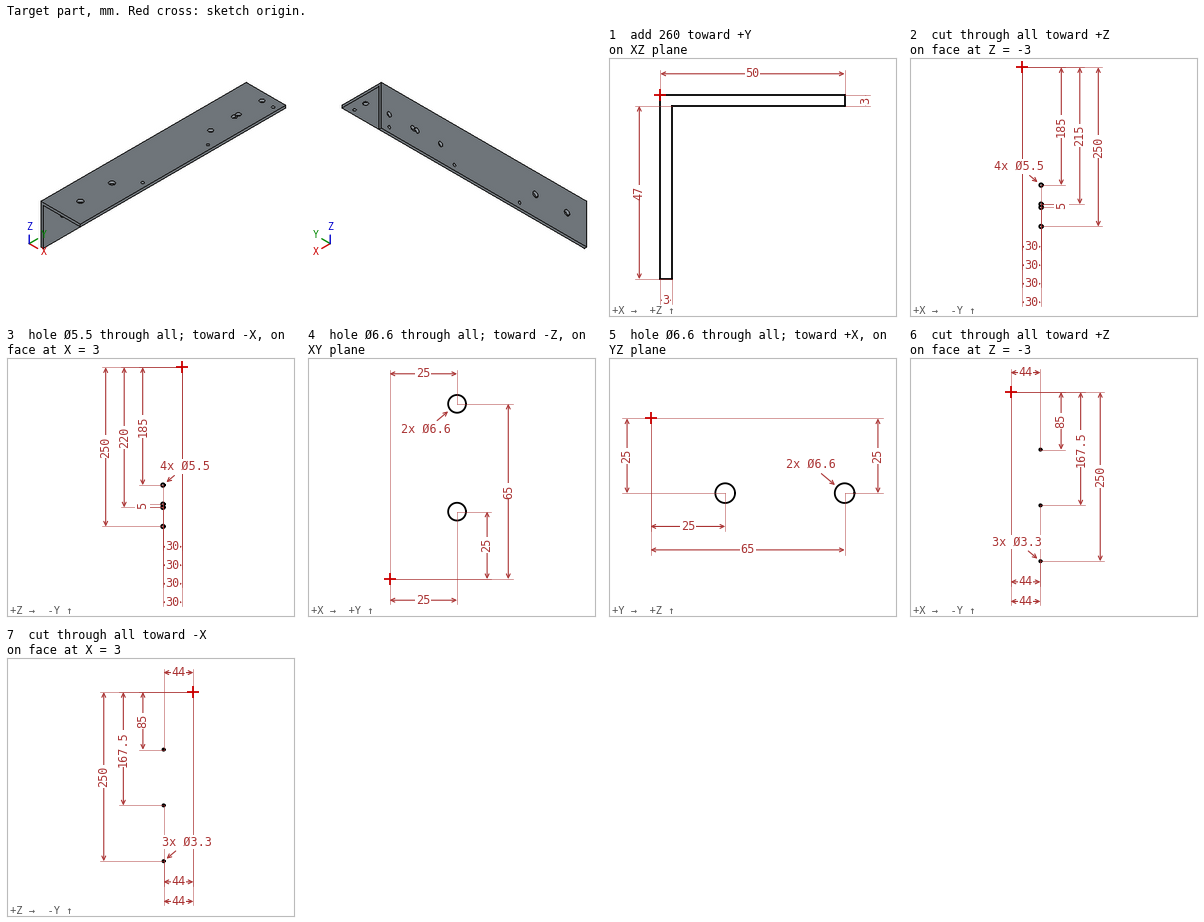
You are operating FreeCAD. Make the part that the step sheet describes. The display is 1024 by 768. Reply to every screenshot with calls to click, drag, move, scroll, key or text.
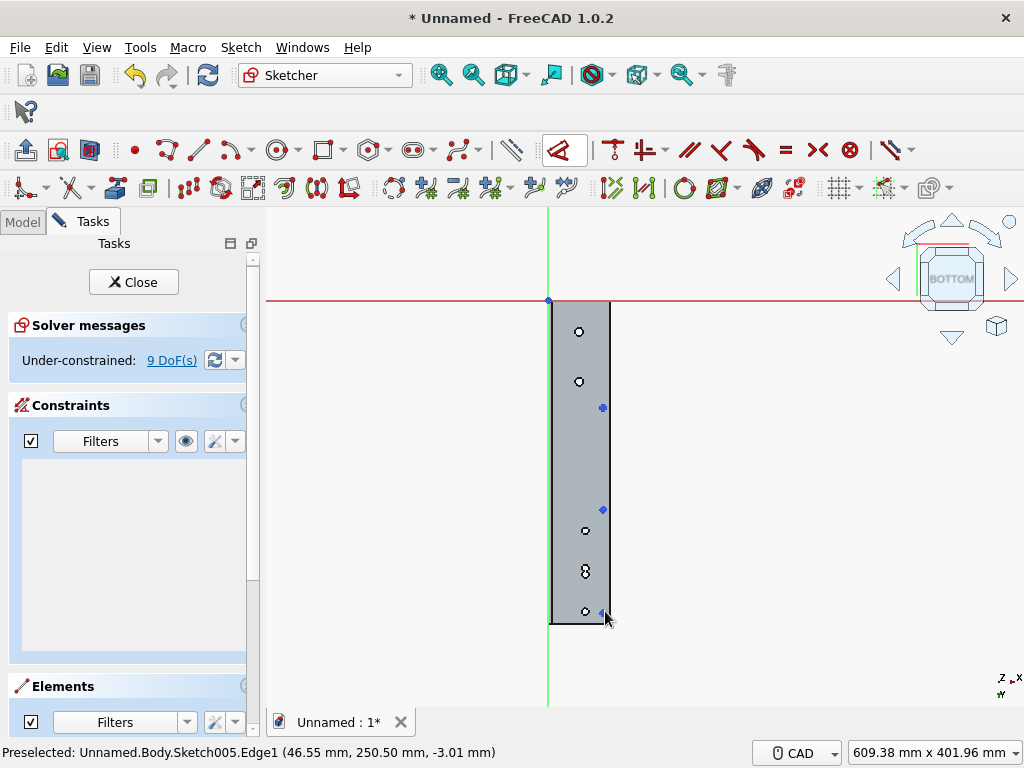
scroll(605, 508, up, 9)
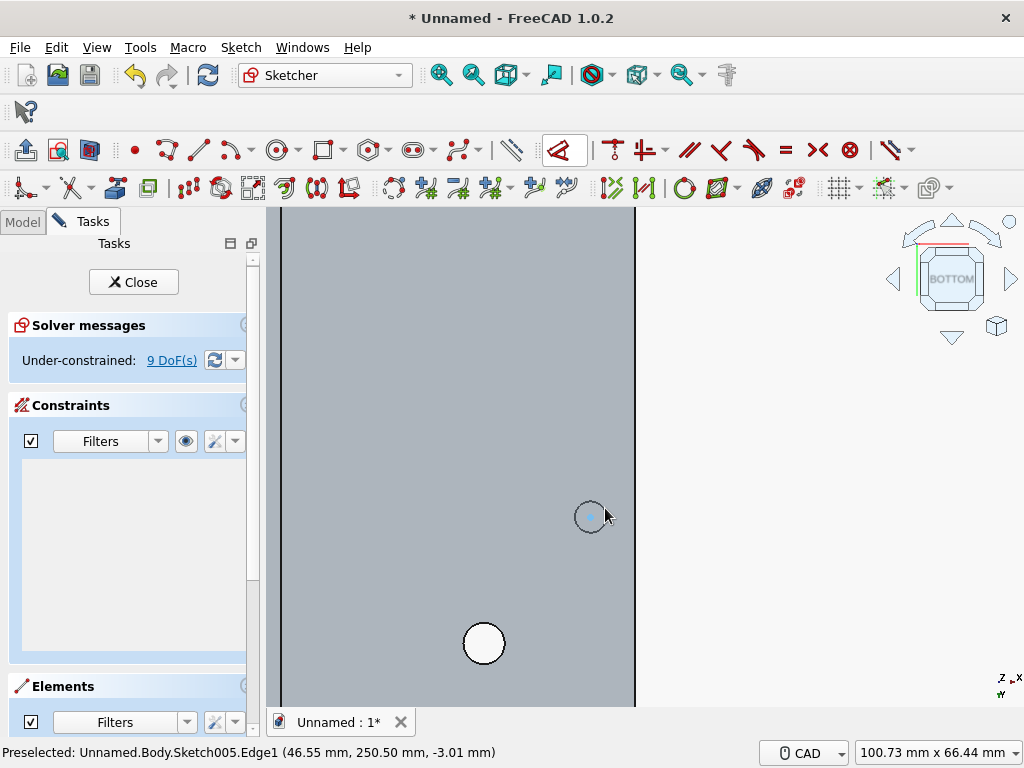
click(602, 506)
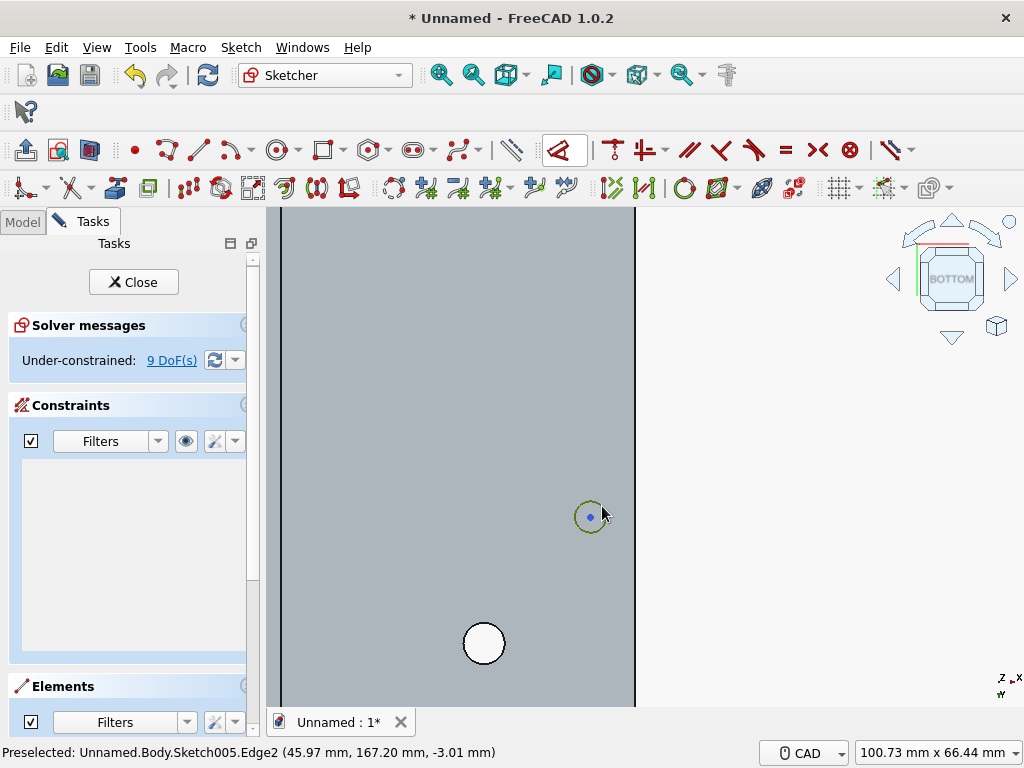
scroll(605, 508, down, 9)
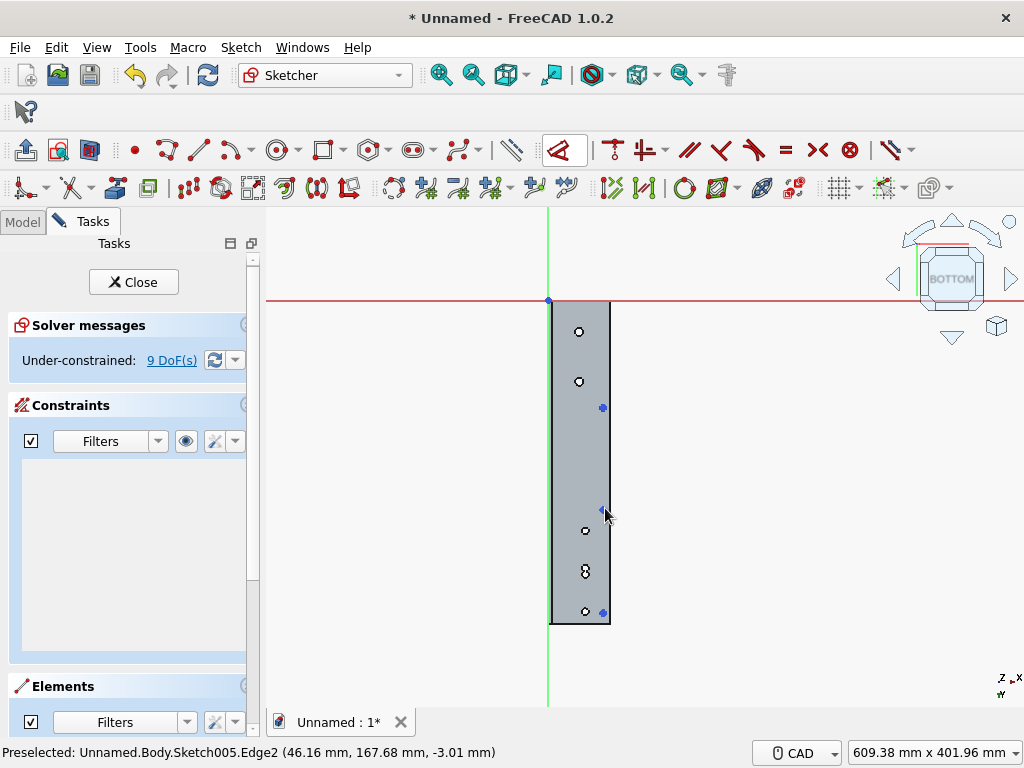
scroll(605, 406, up, 8)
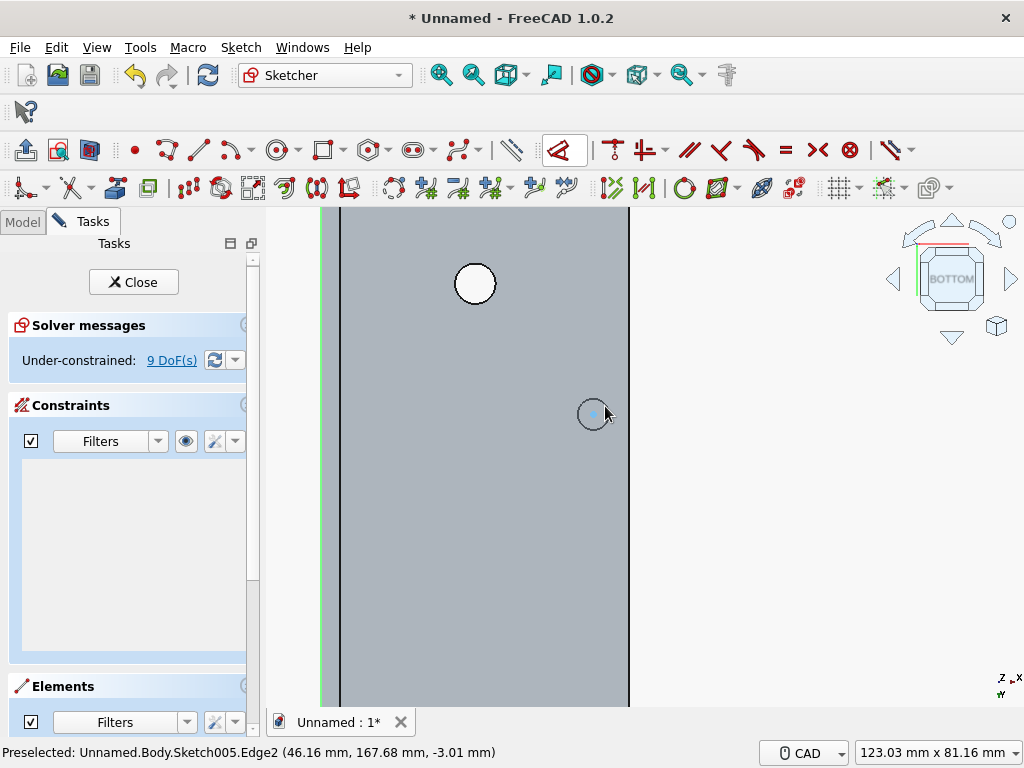
click(604, 403)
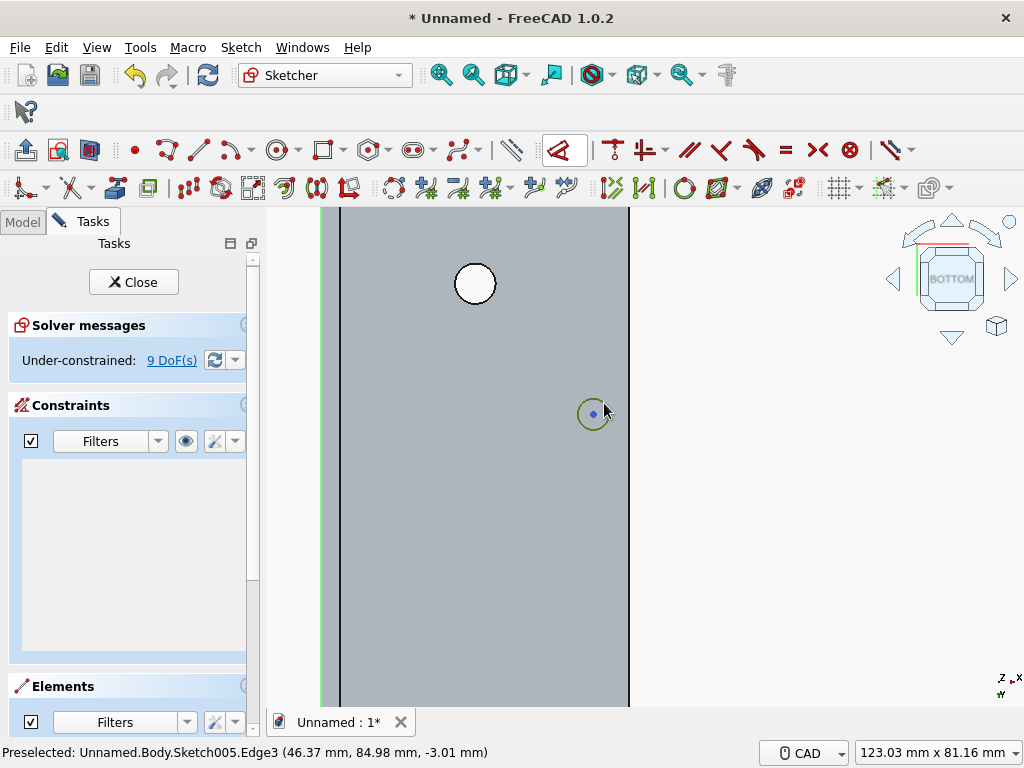
click(786, 150)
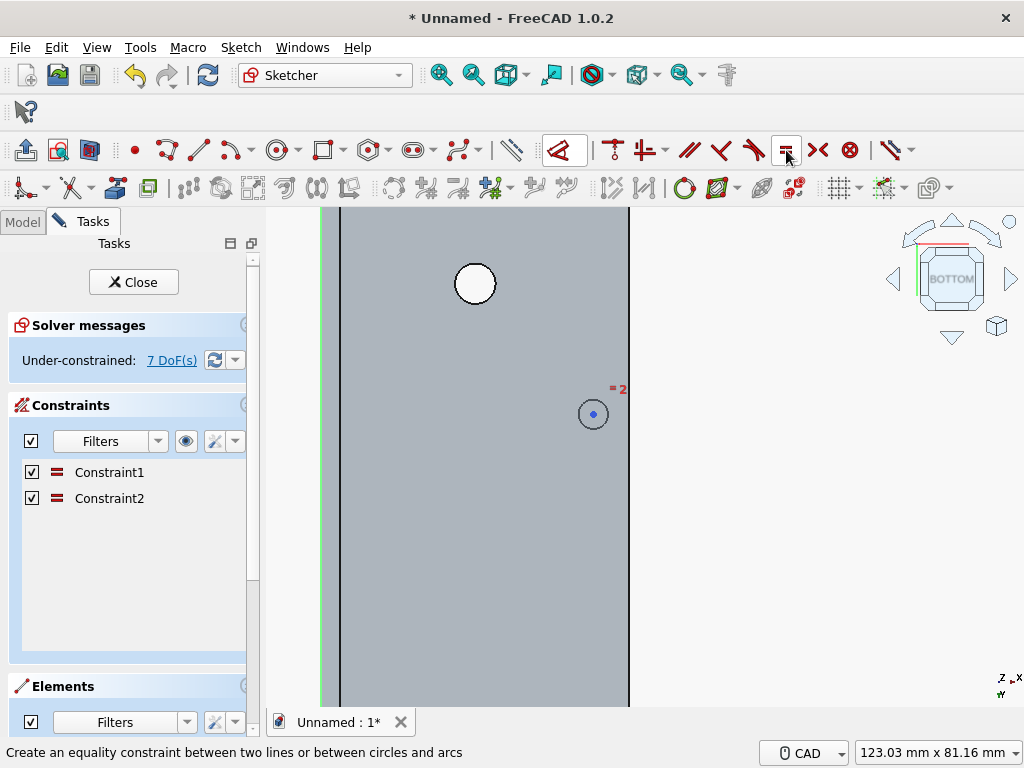
scroll(605, 406, down, 8)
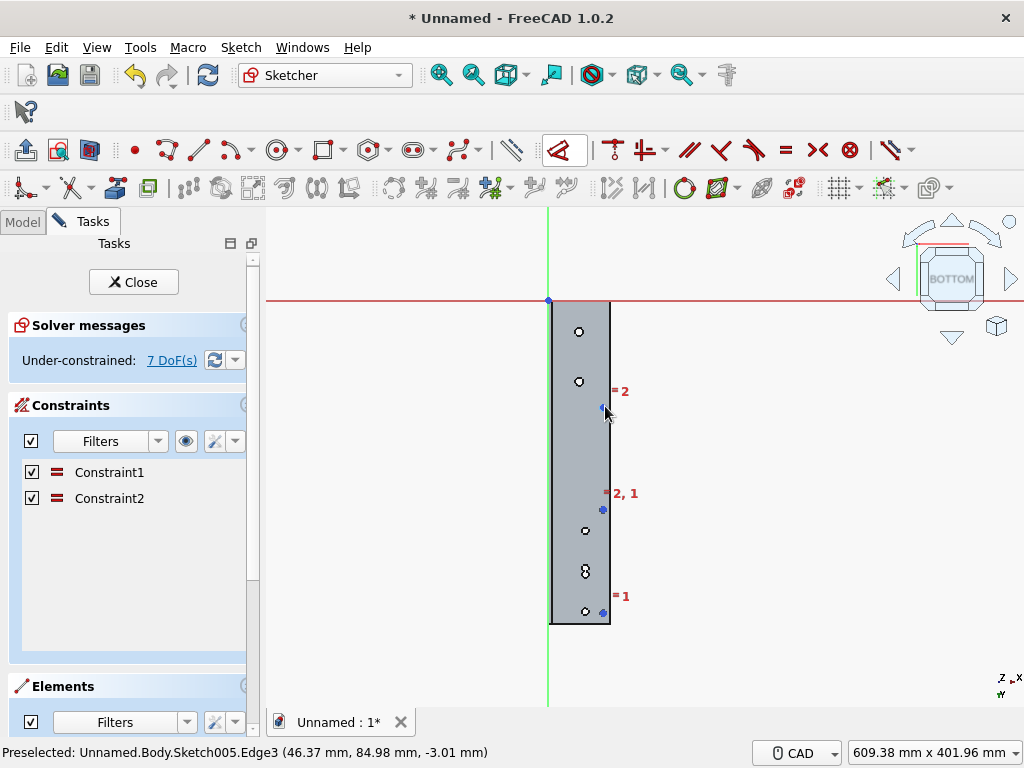
scroll(605, 611, up, 12)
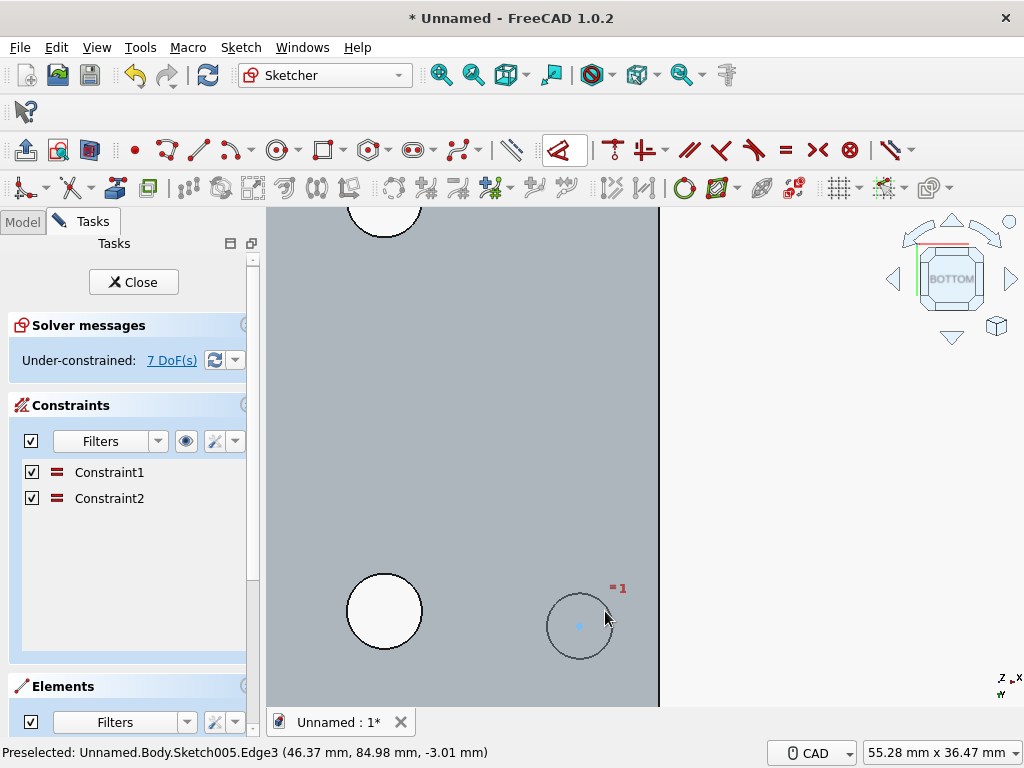
click(603, 603)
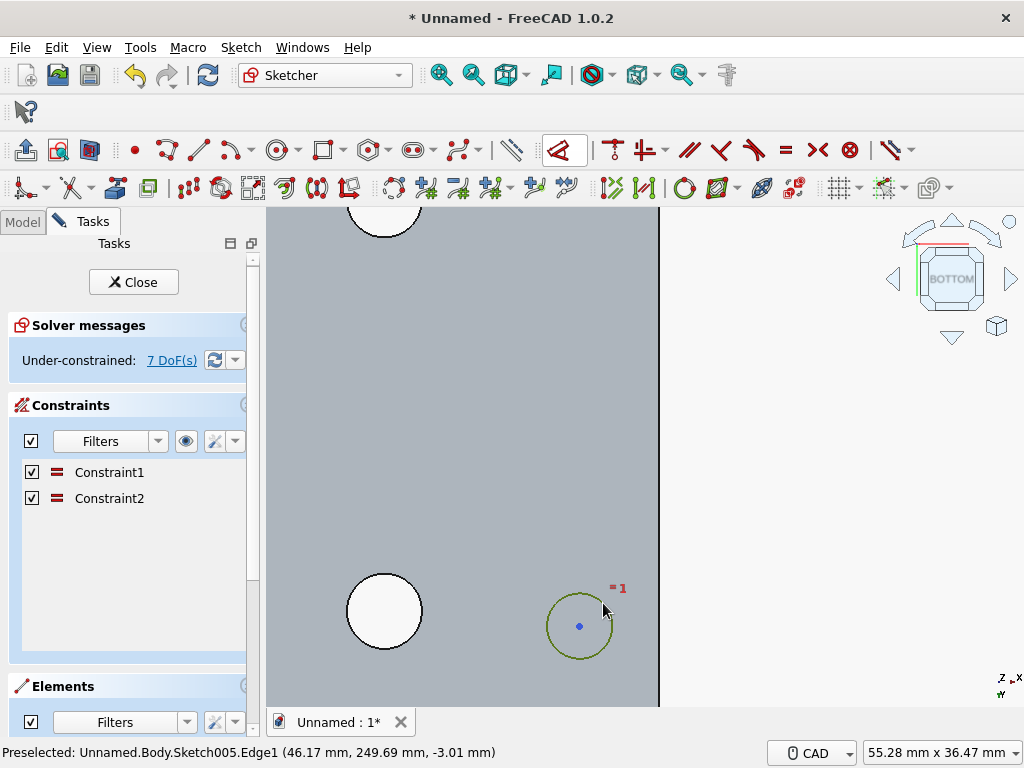
click(582, 150)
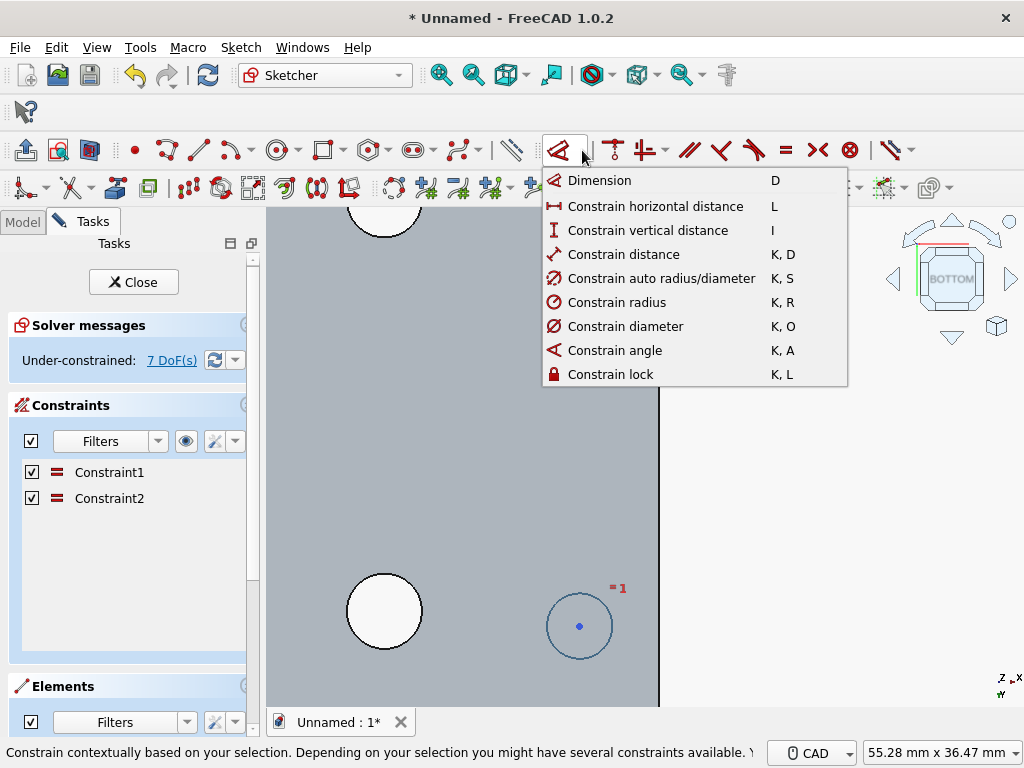
click(695, 326)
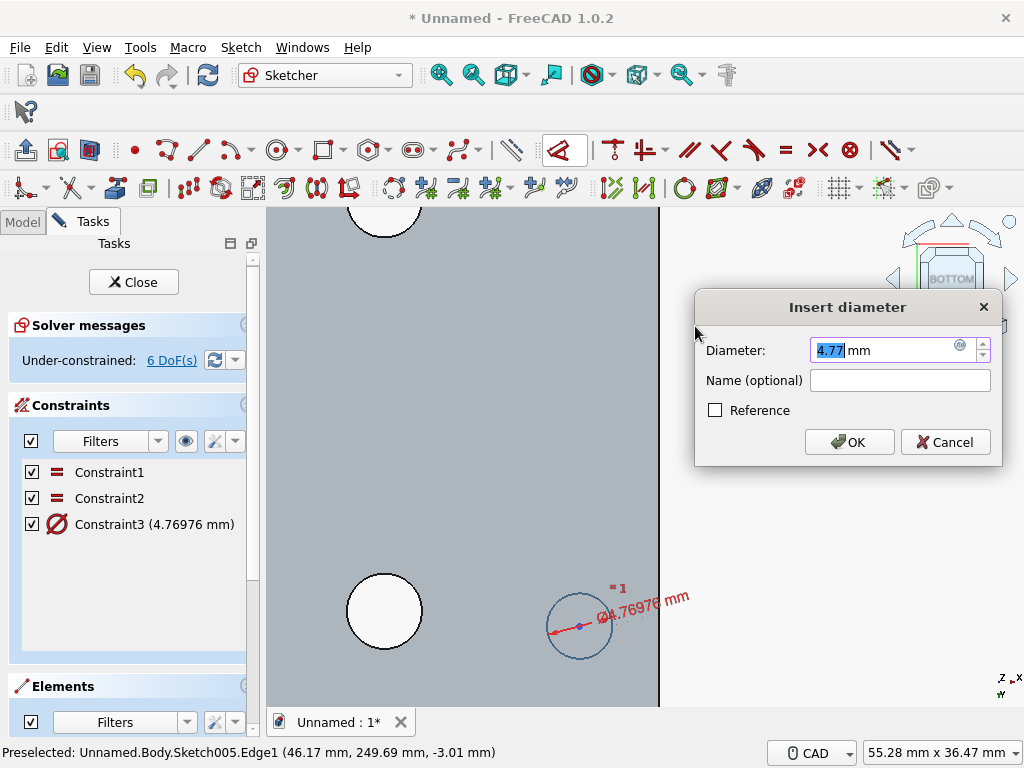
text(3.3)
key(Return)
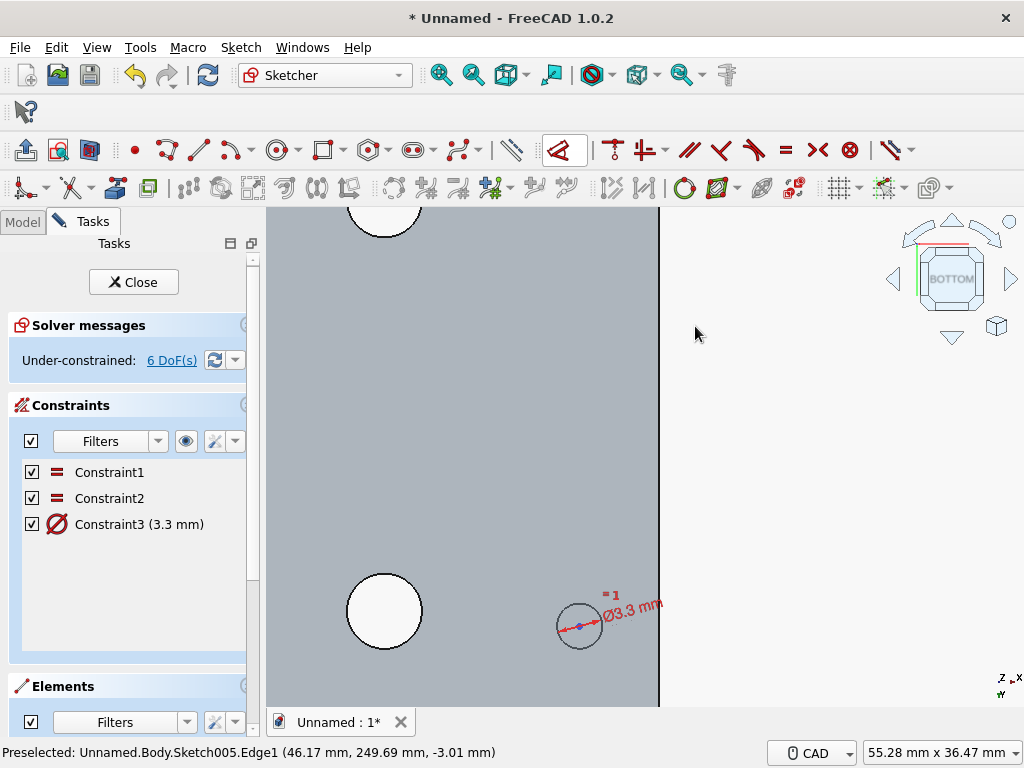
scroll(605, 611, down, 12)